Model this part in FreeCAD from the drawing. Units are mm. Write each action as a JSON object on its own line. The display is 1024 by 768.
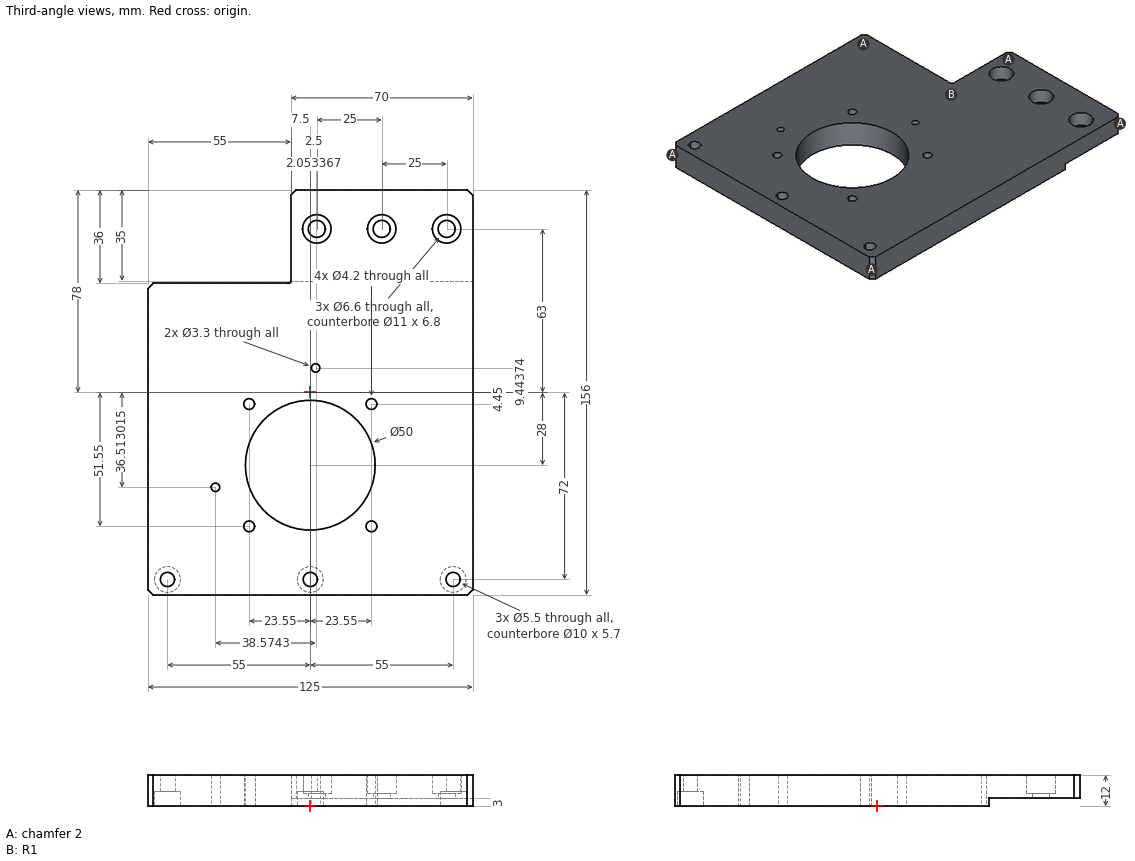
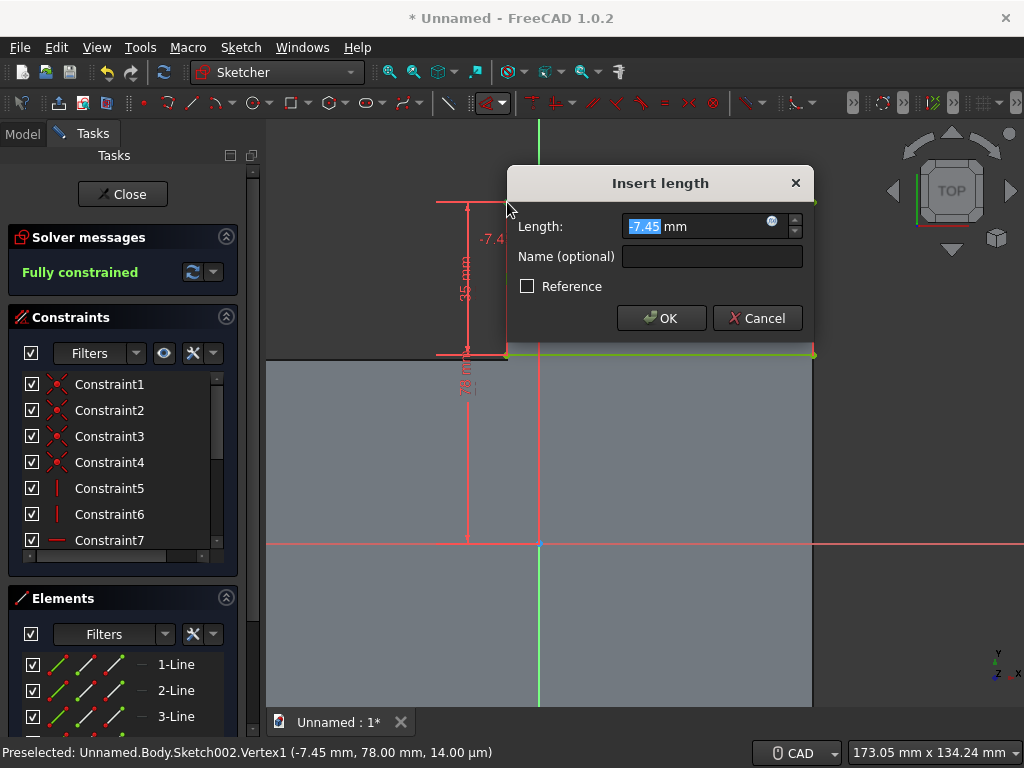
{"action": "type", "text": "-7.5"}
{"action": "key", "text": "Return"}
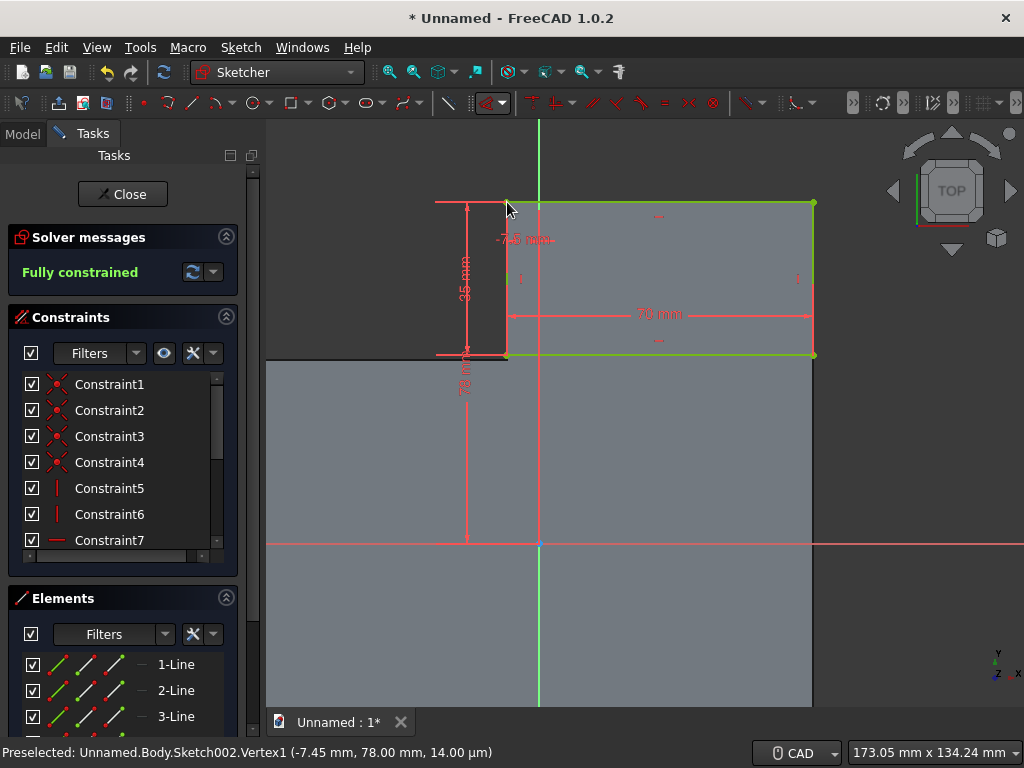
{"action": "left_click", "coordinate": [123, 194]}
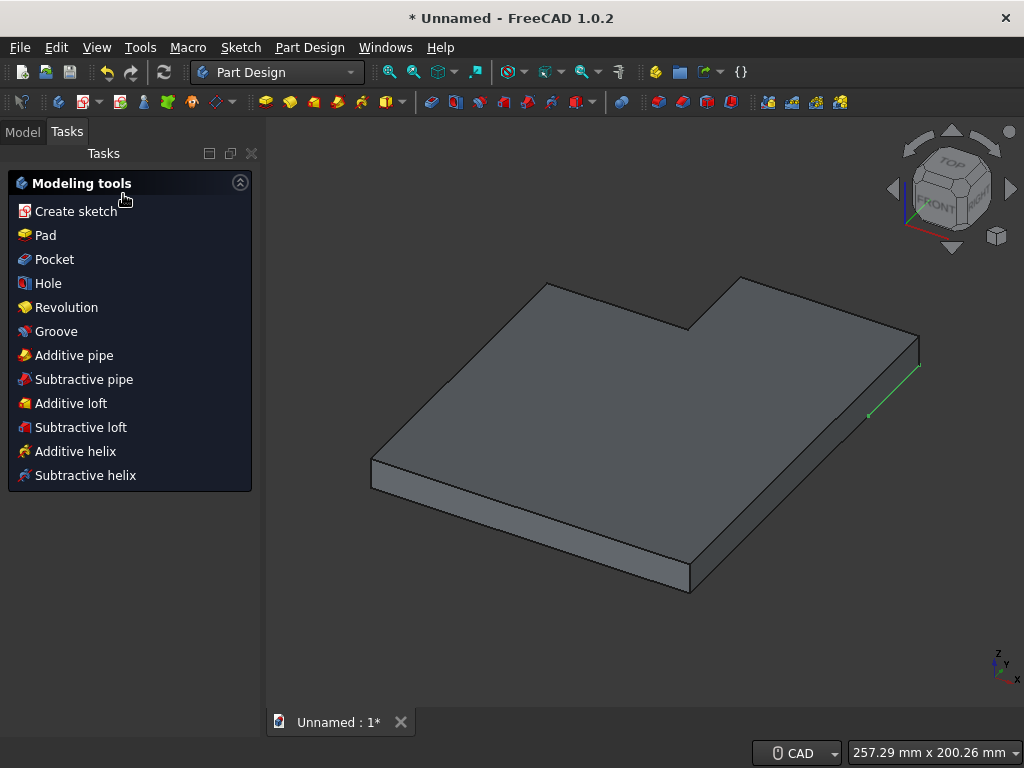
{"action": "left_click", "coordinate": [432, 102]}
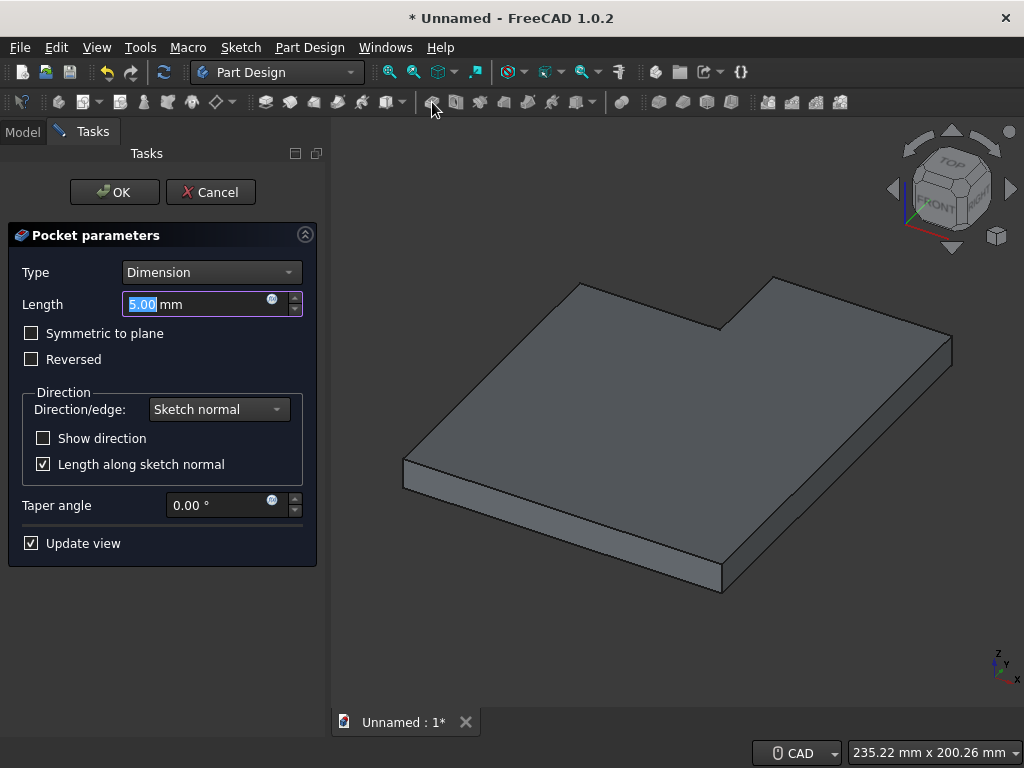
{"action": "type", "text": "3"}
{"action": "key", "text": "Tab"}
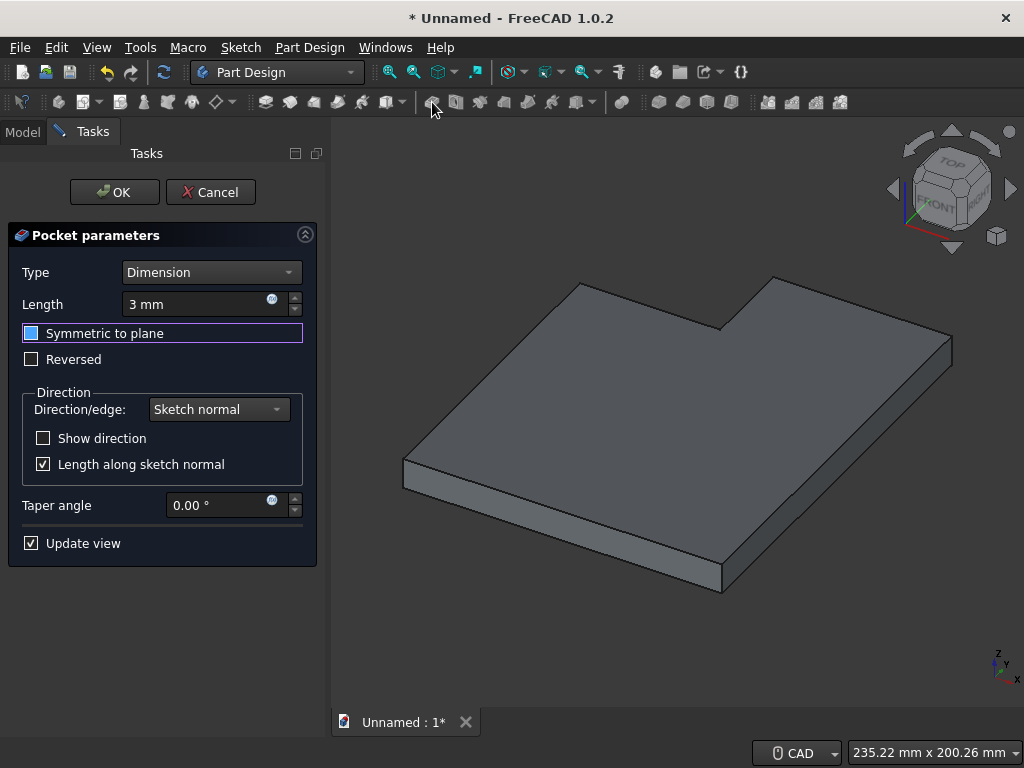
{"action": "left_click", "coordinate": [30, 359]}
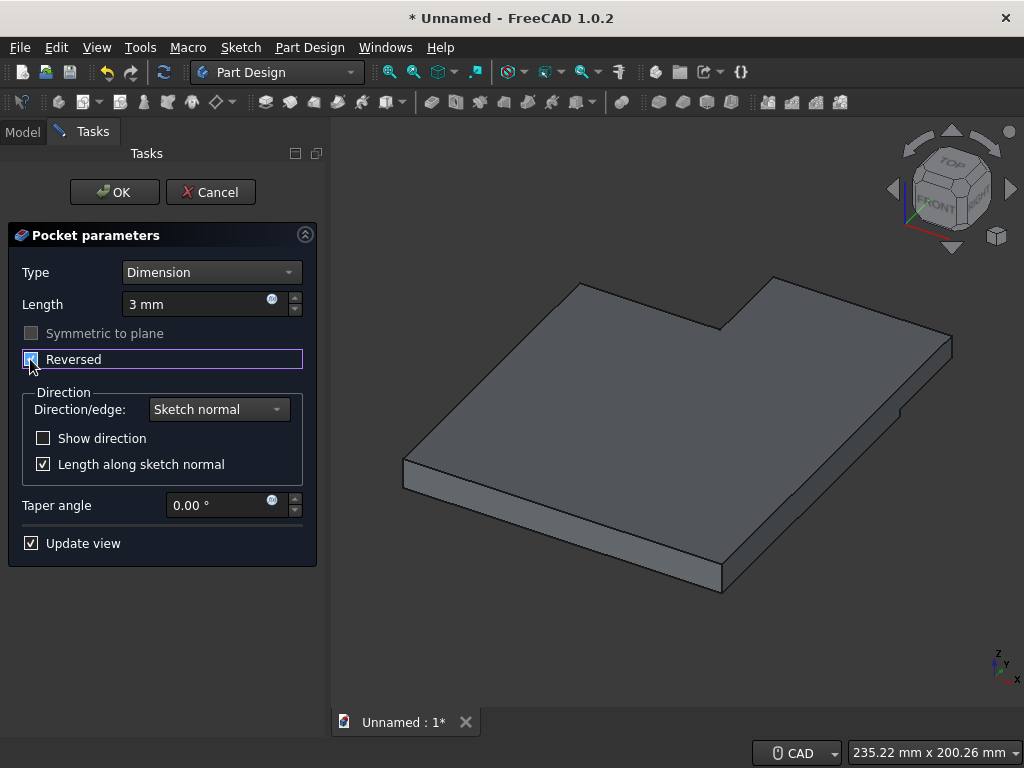
{"action": "left_click", "coordinate": [115, 192]}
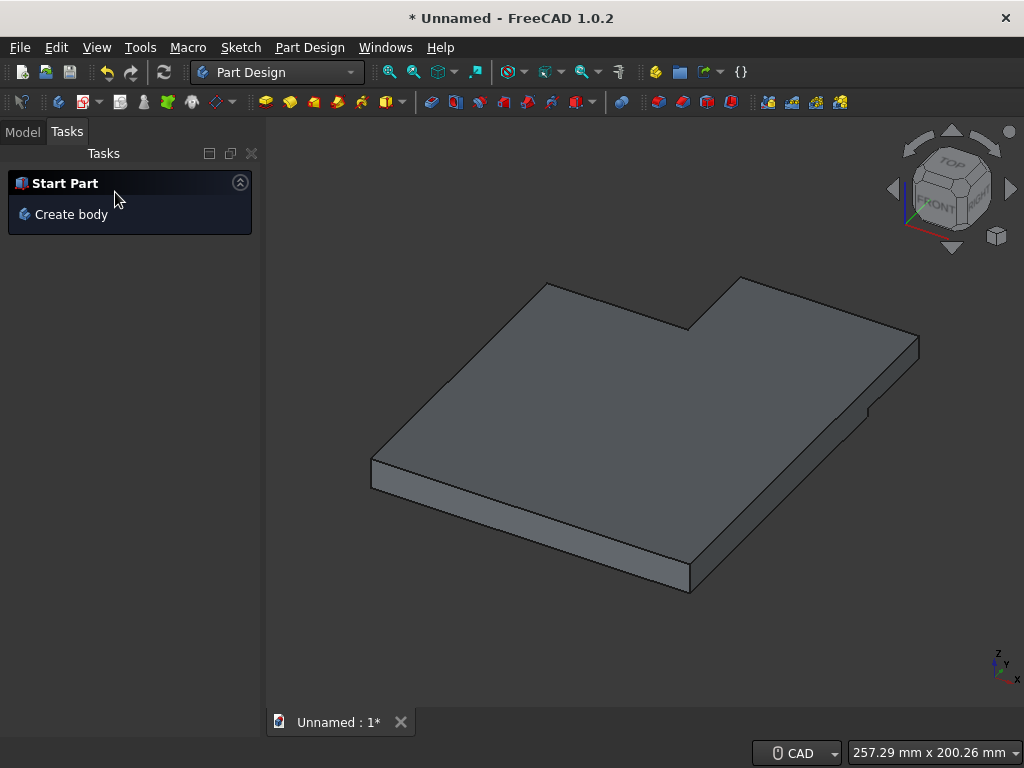
{"action": "key", "text": "5"}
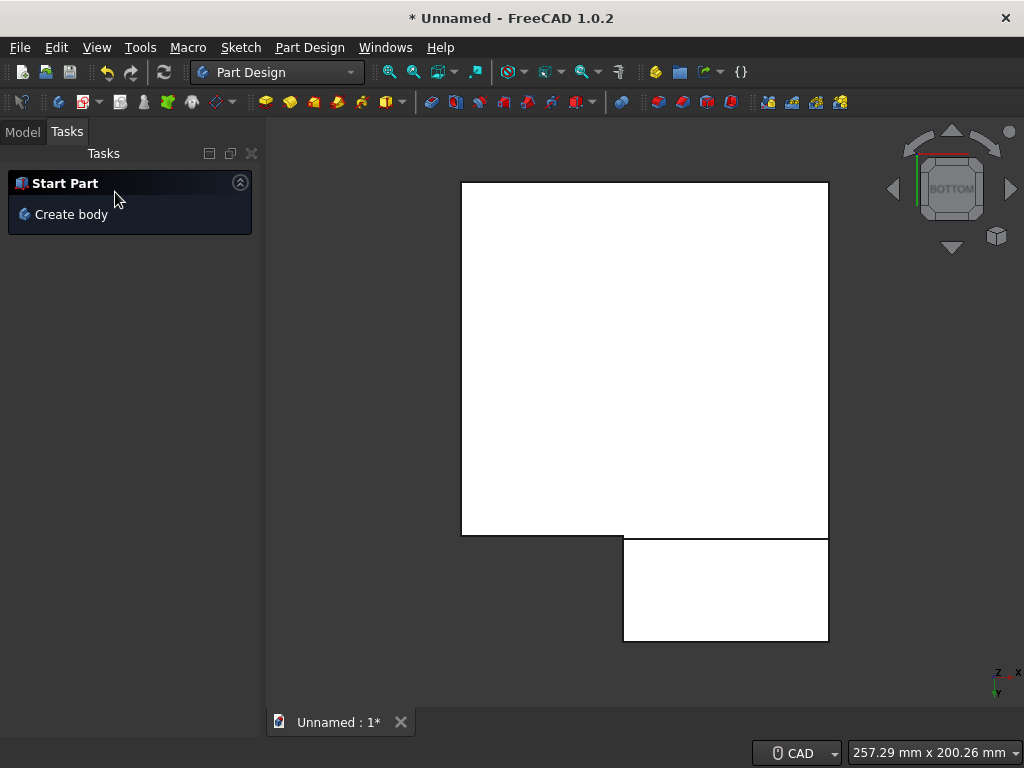
{"action": "left_click", "coordinate": [645, 359]}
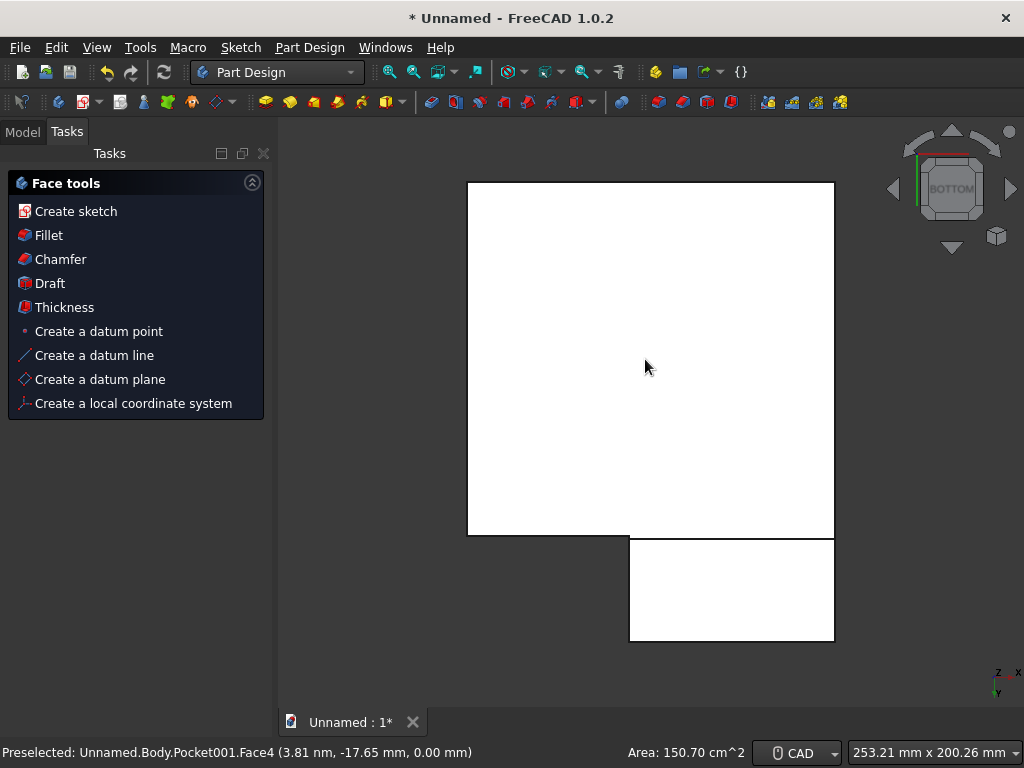
{"action": "left_click", "coordinate": [84, 102]}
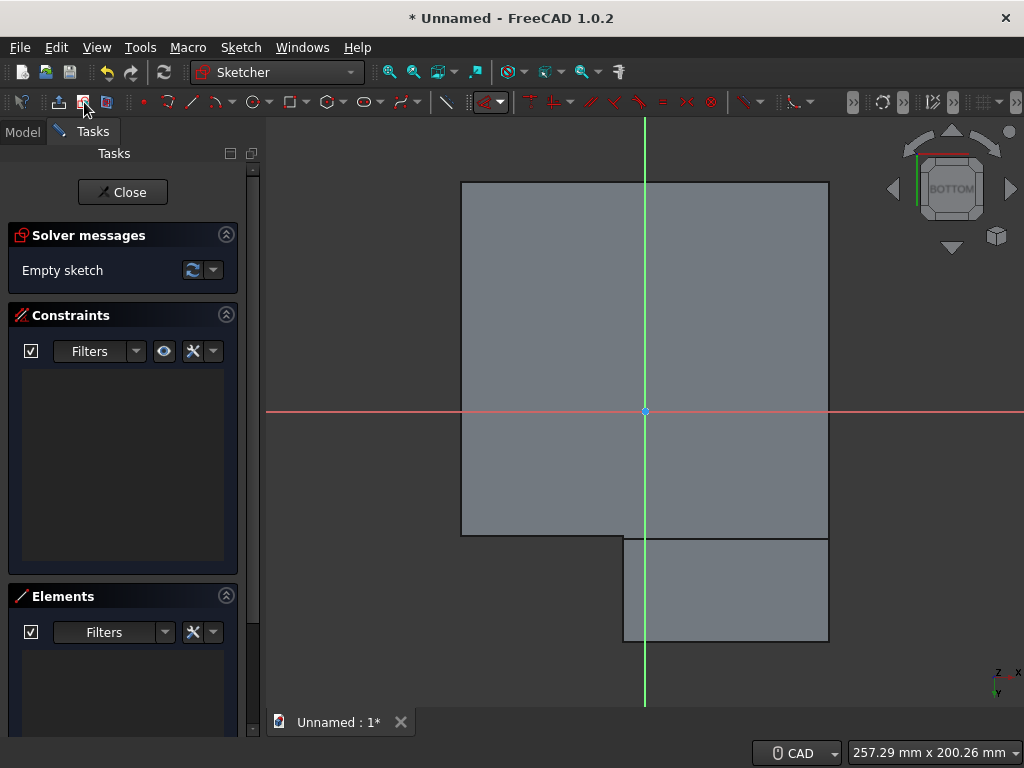
{"action": "left_click", "coordinate": [254, 102]}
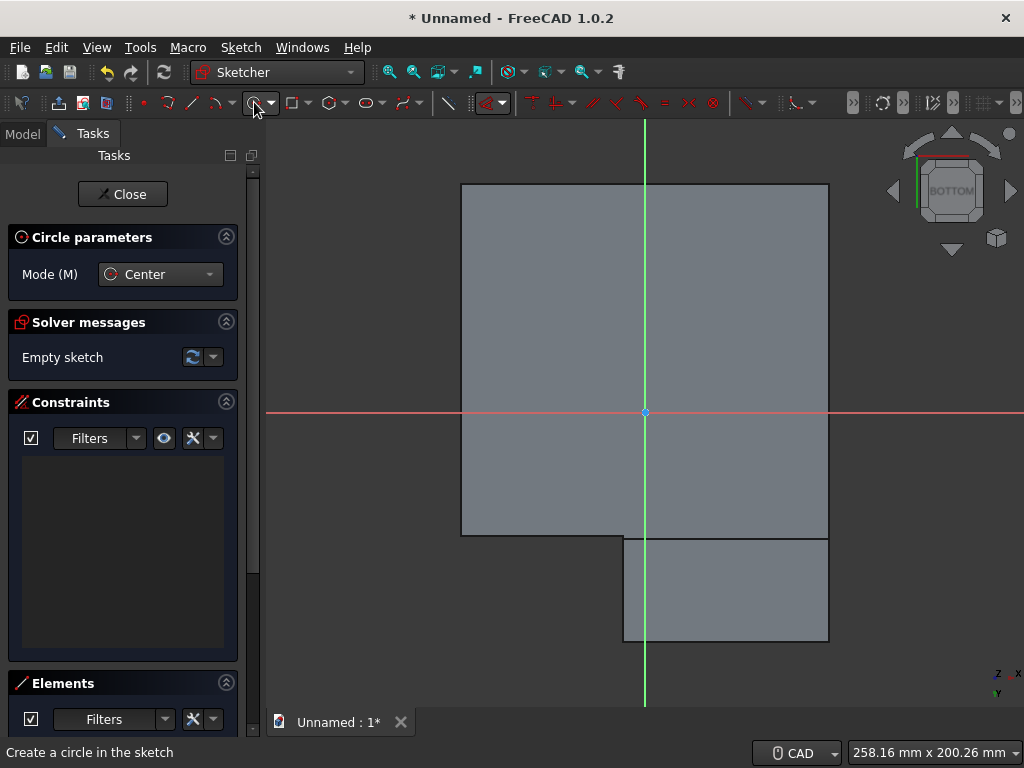
{"action": "scroll", "coordinate": [806, 202], "scroll_direction": "up", "scroll_amount": 6}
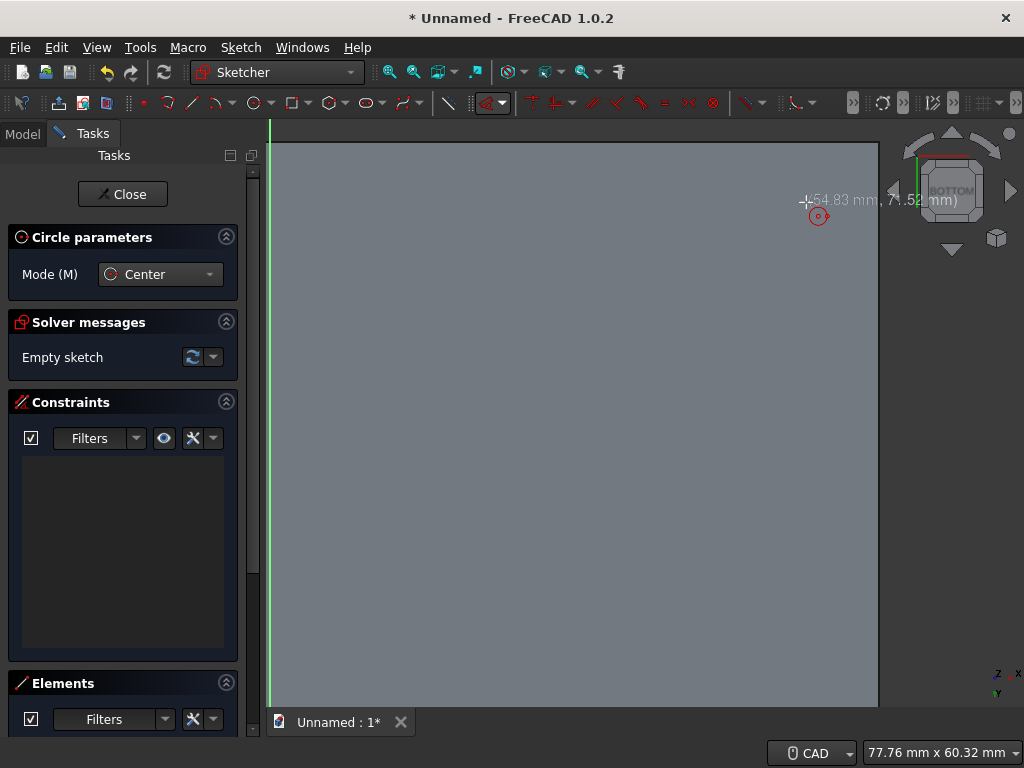
{"action": "left_click", "coordinate": [806, 200]}
{"action": "left_click", "coordinate": [825, 181]}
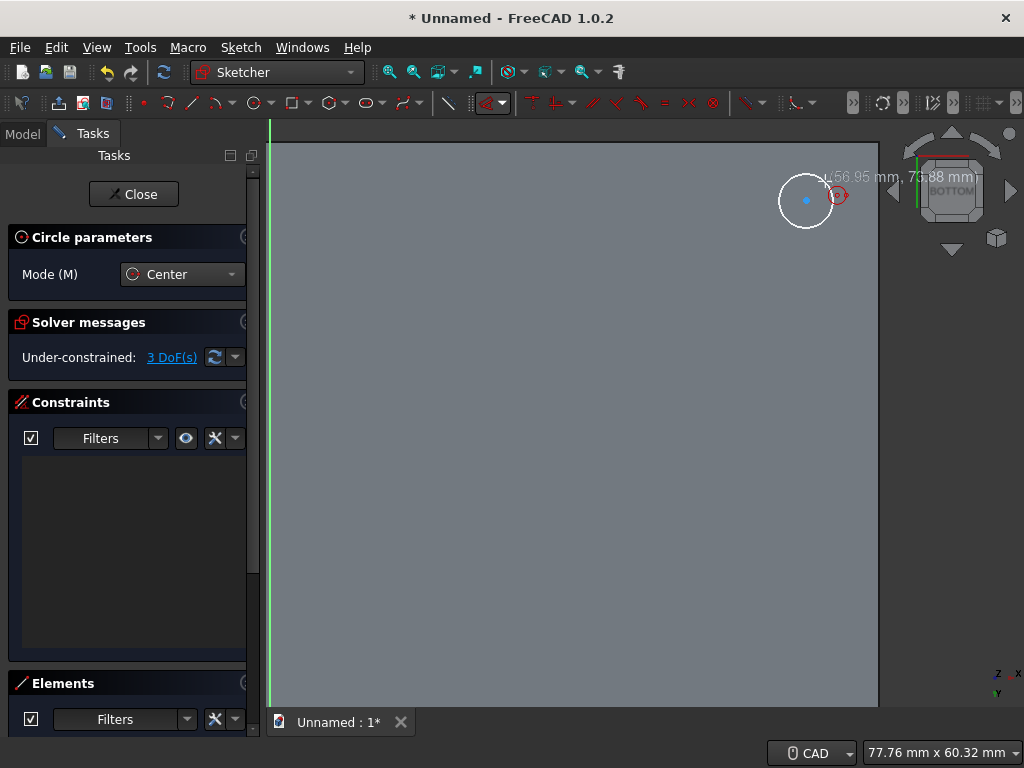
{"action": "scroll", "coordinate": [755, 340], "scroll_direction": "down", "scroll_amount": 5}